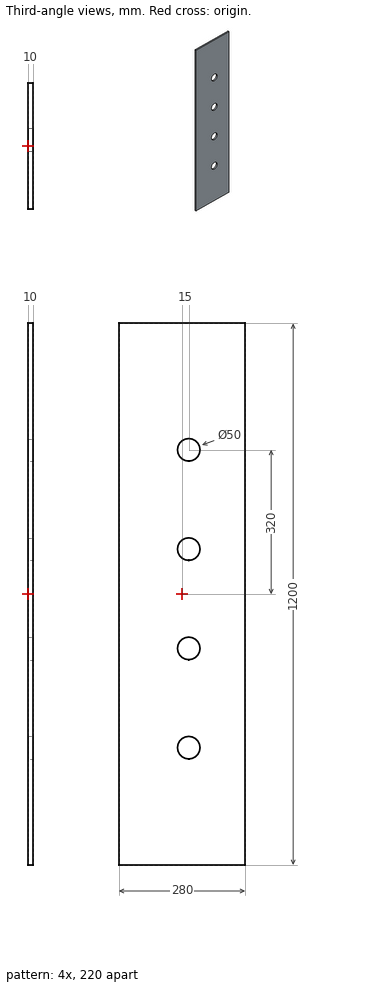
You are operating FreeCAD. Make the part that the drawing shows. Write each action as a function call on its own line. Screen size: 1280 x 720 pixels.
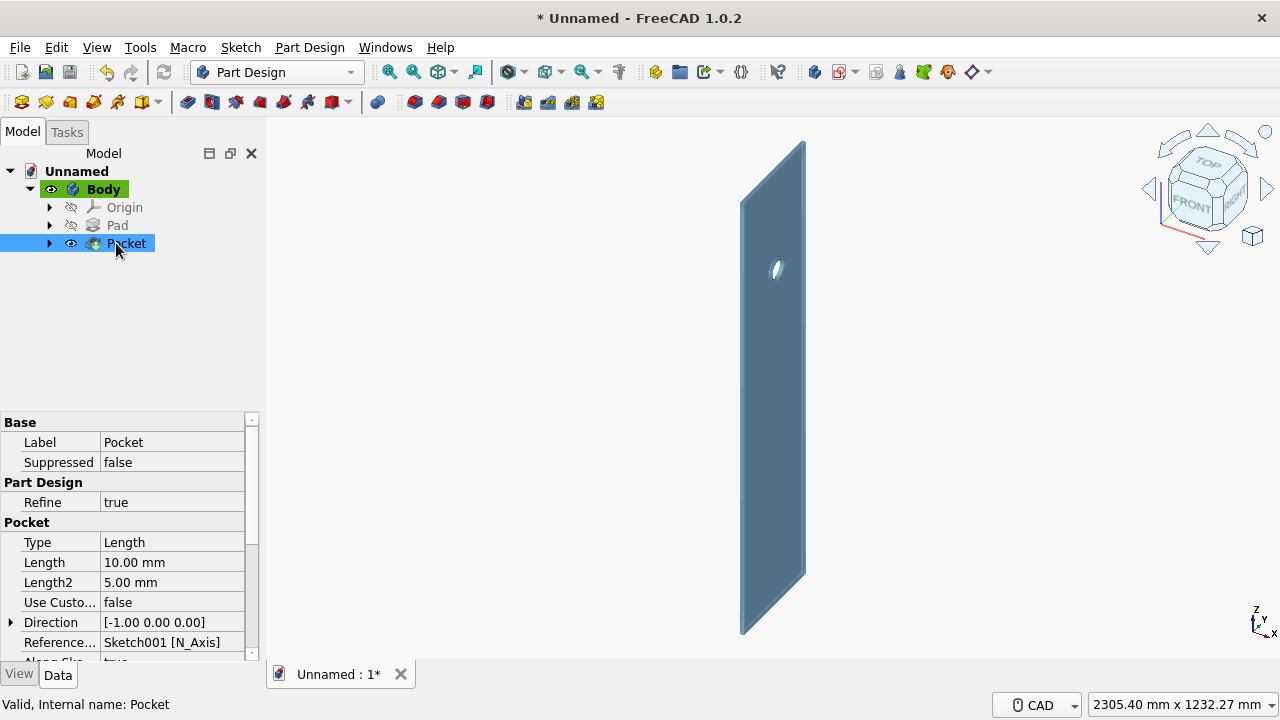
click(548, 102)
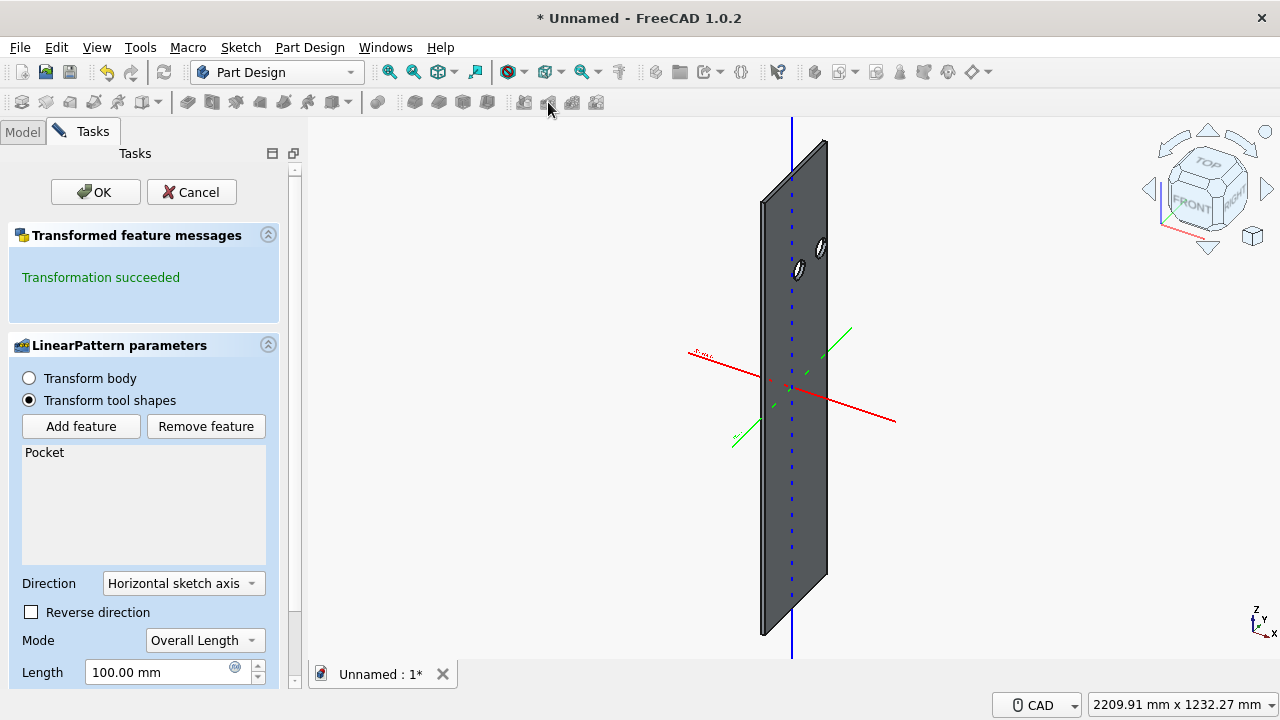
click(184, 584)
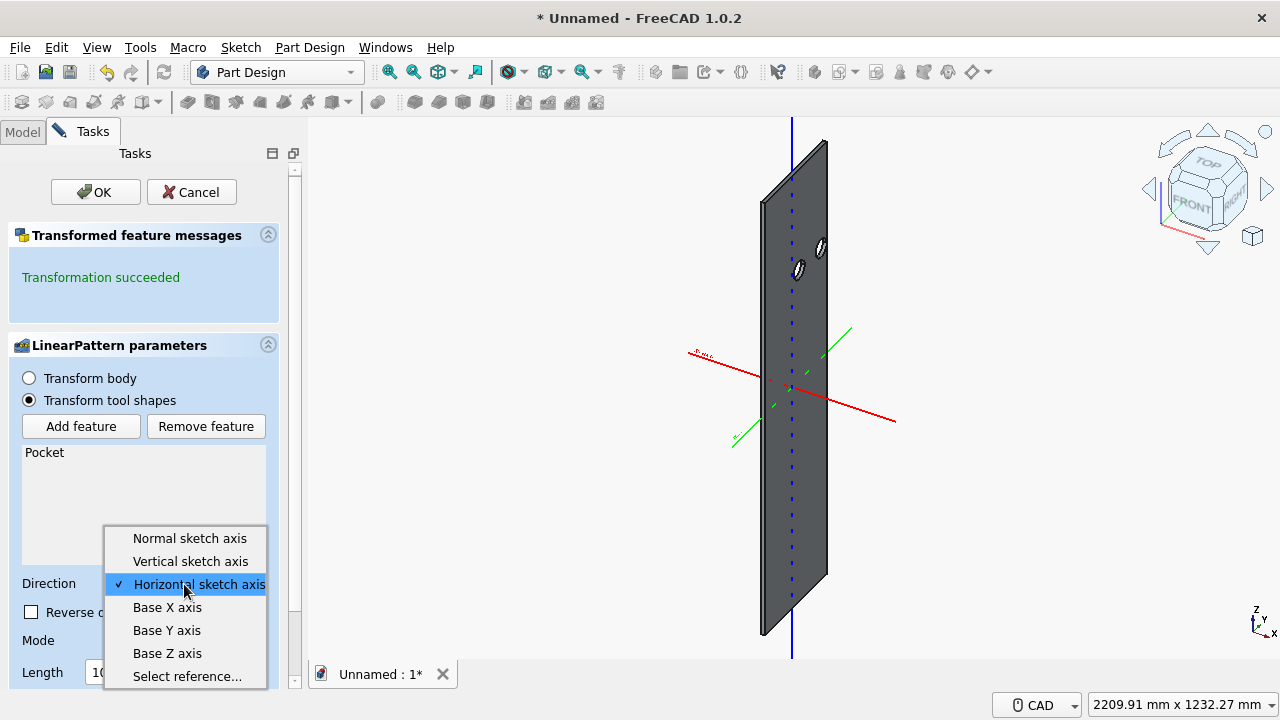
click(184, 654)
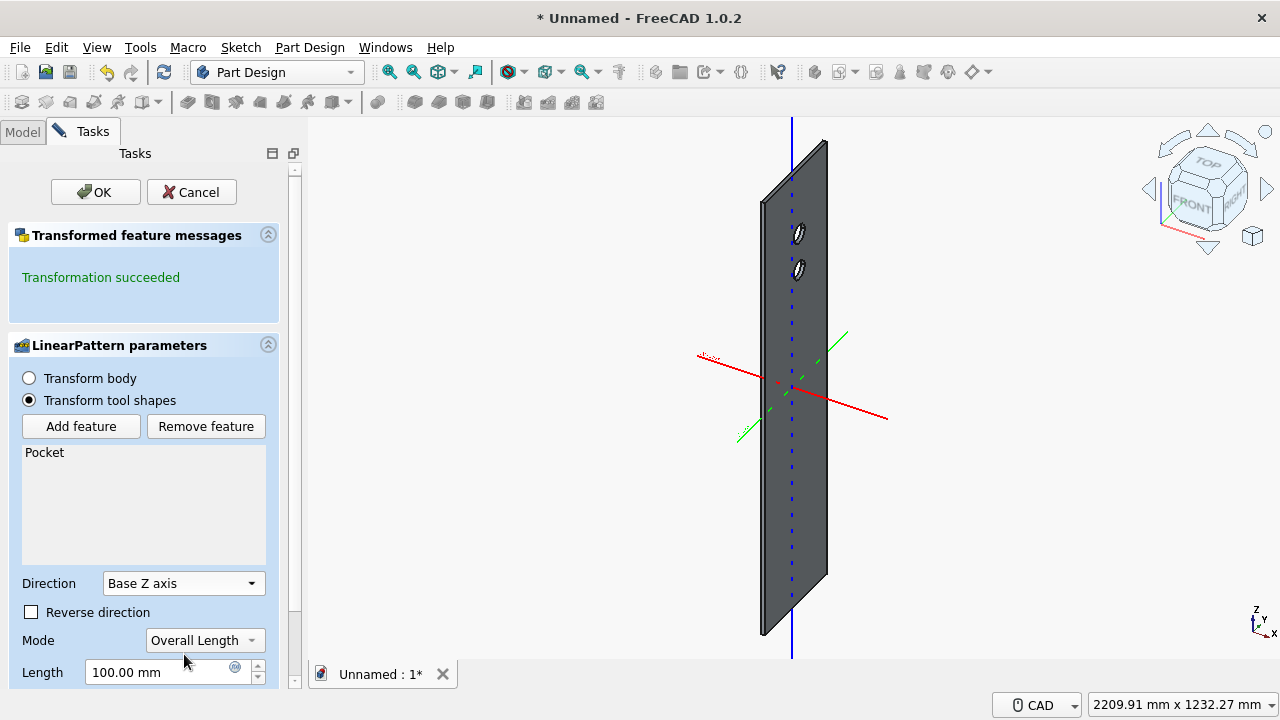
click(206, 640)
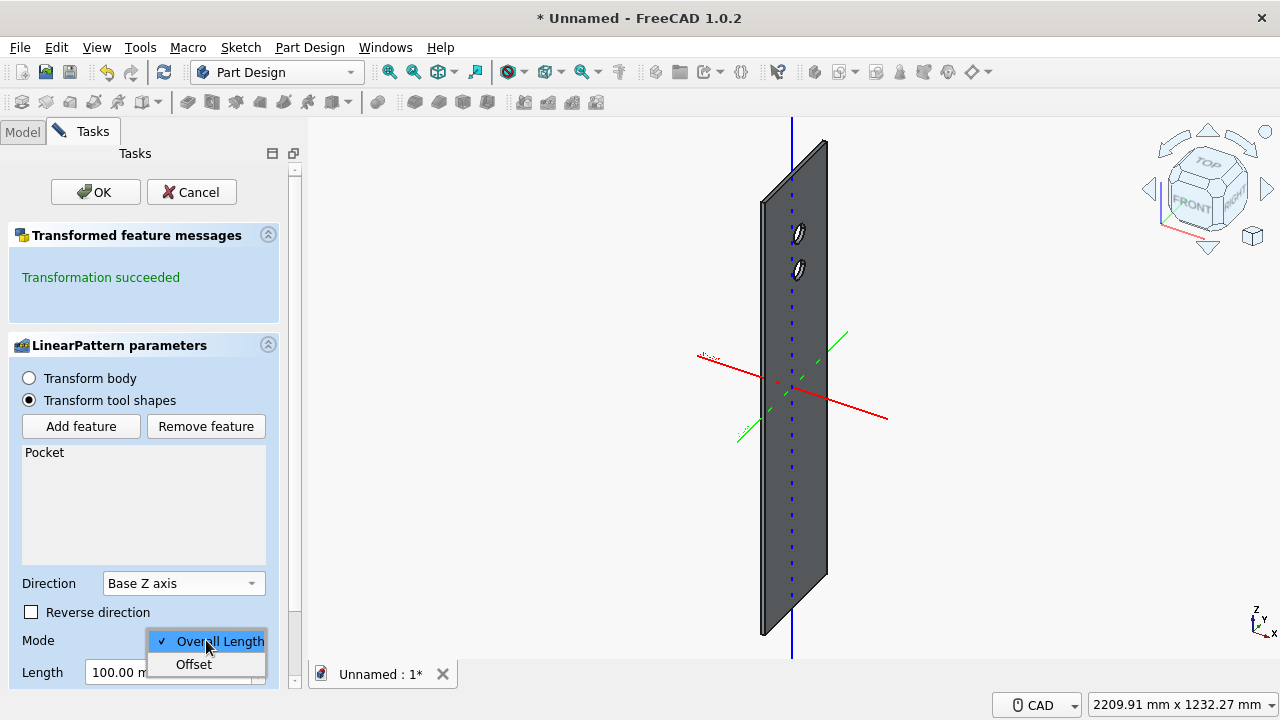
click(206, 664)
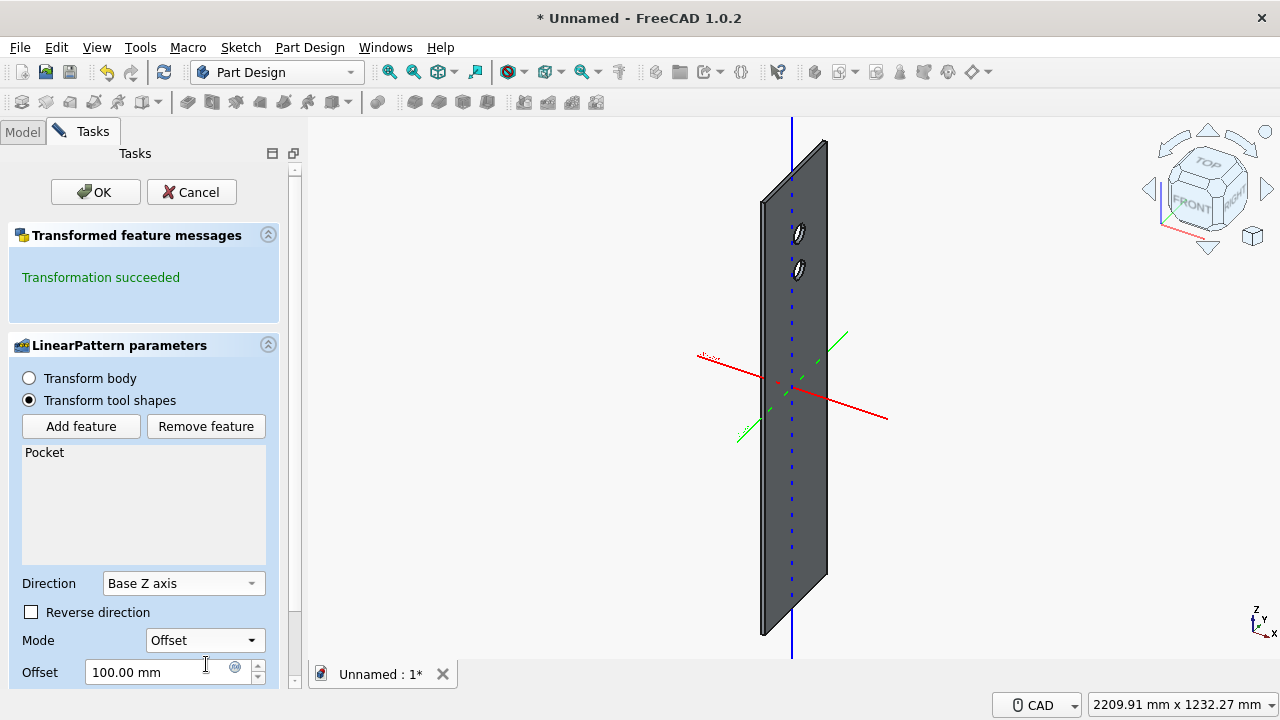
triple_click(168, 672)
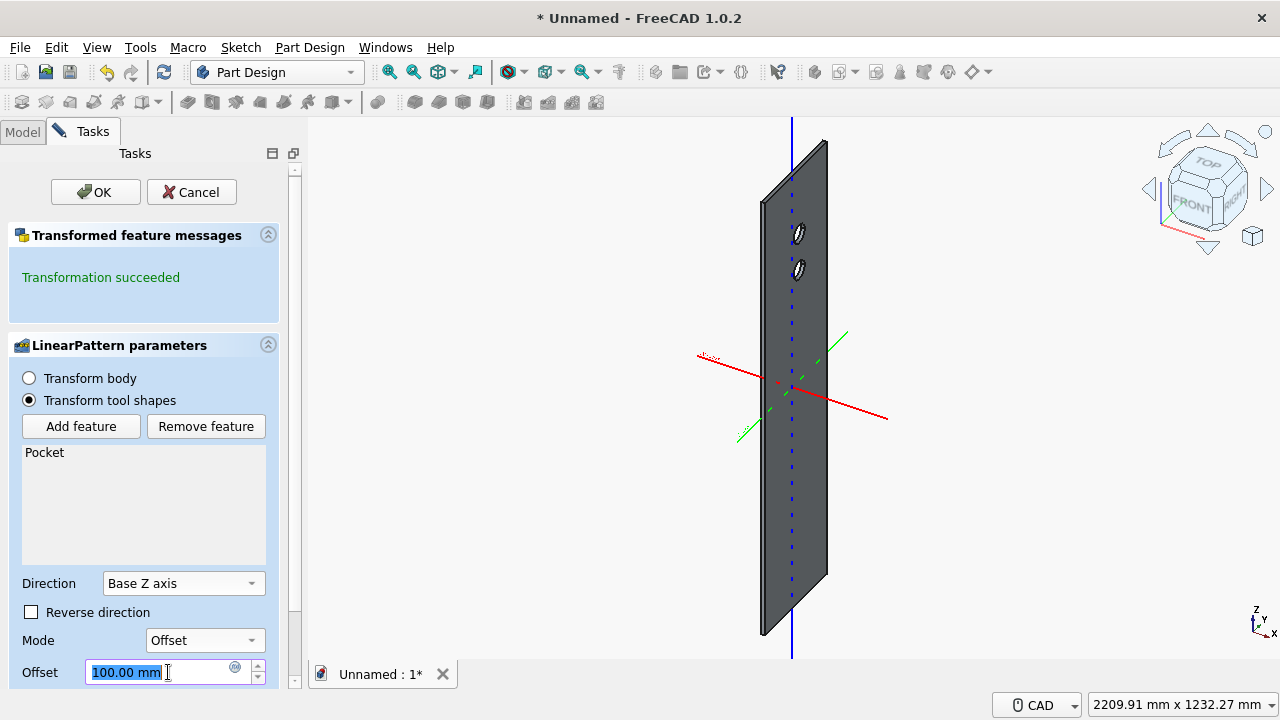
text(220)
key(Tab)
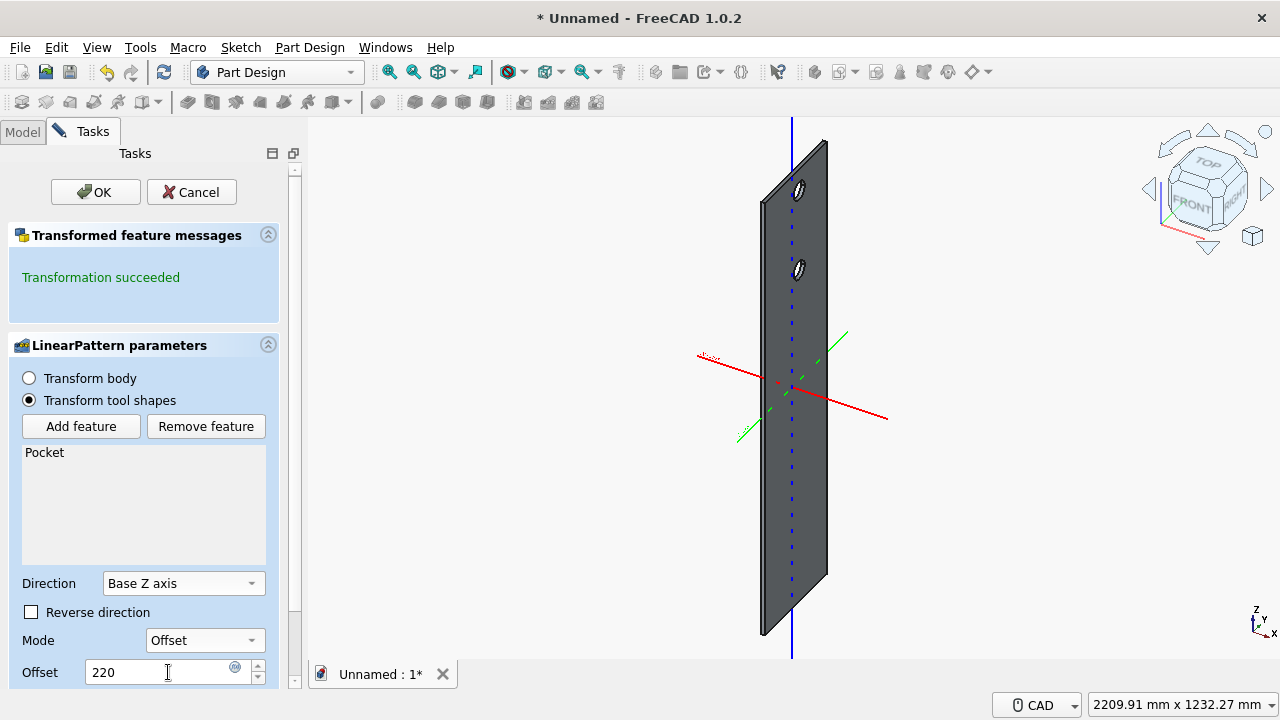
scroll(295, 426, down, 2)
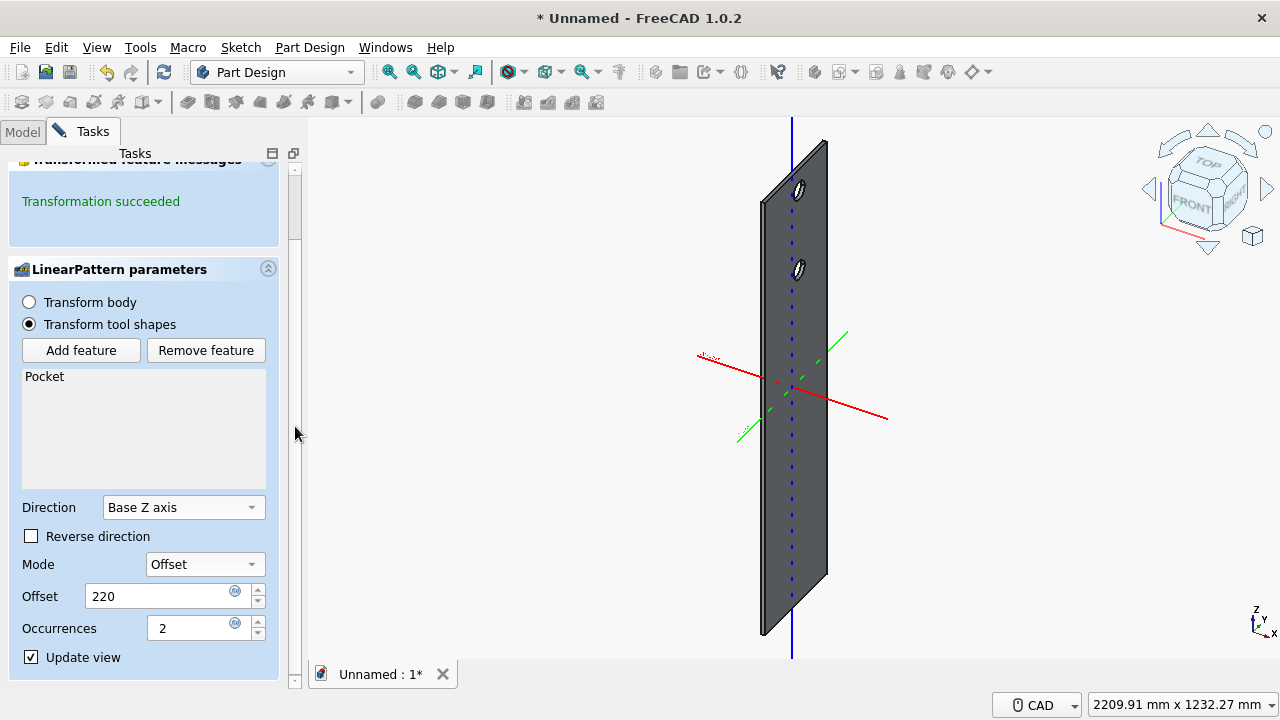
triple_click(198, 628)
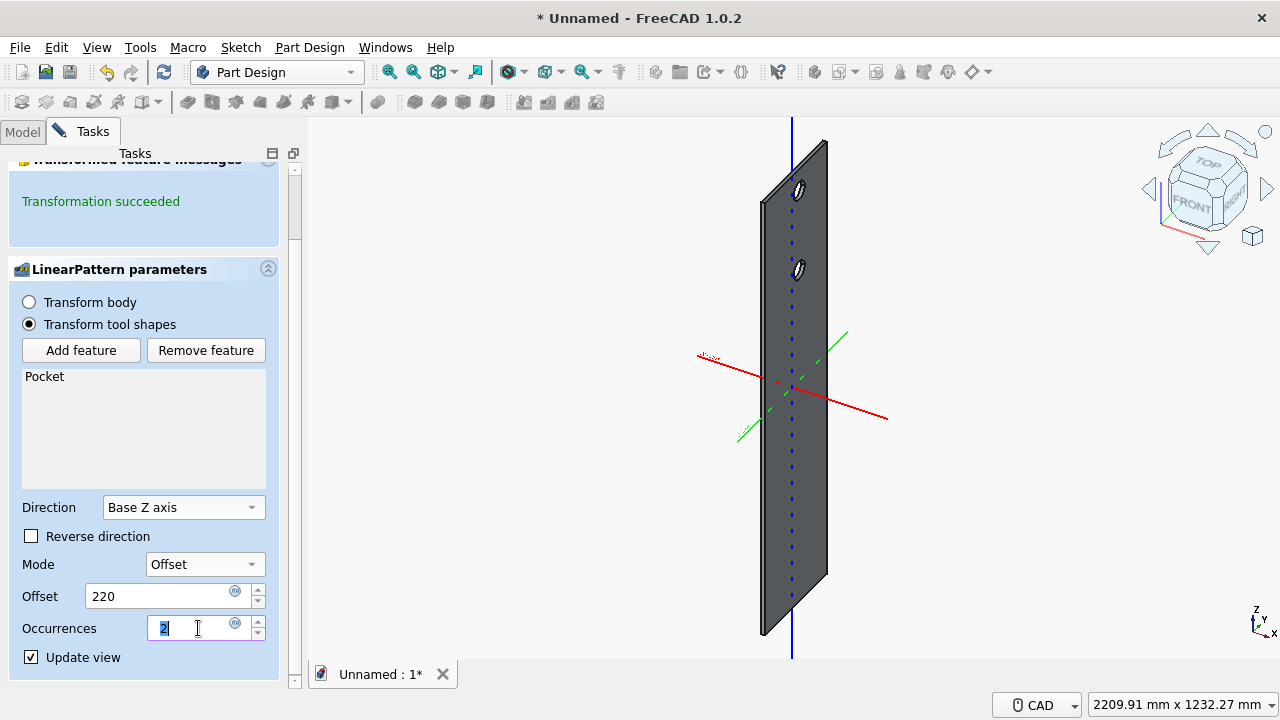
text(4)
key(Tab)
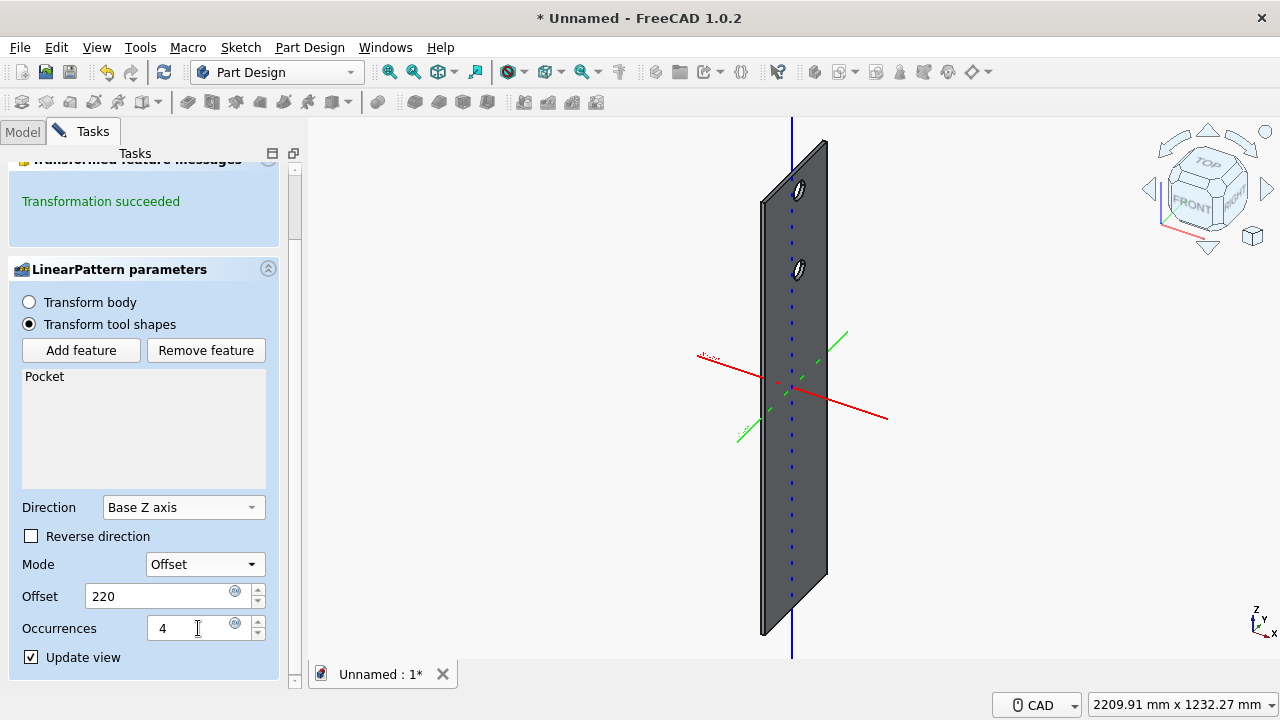
click(30, 536)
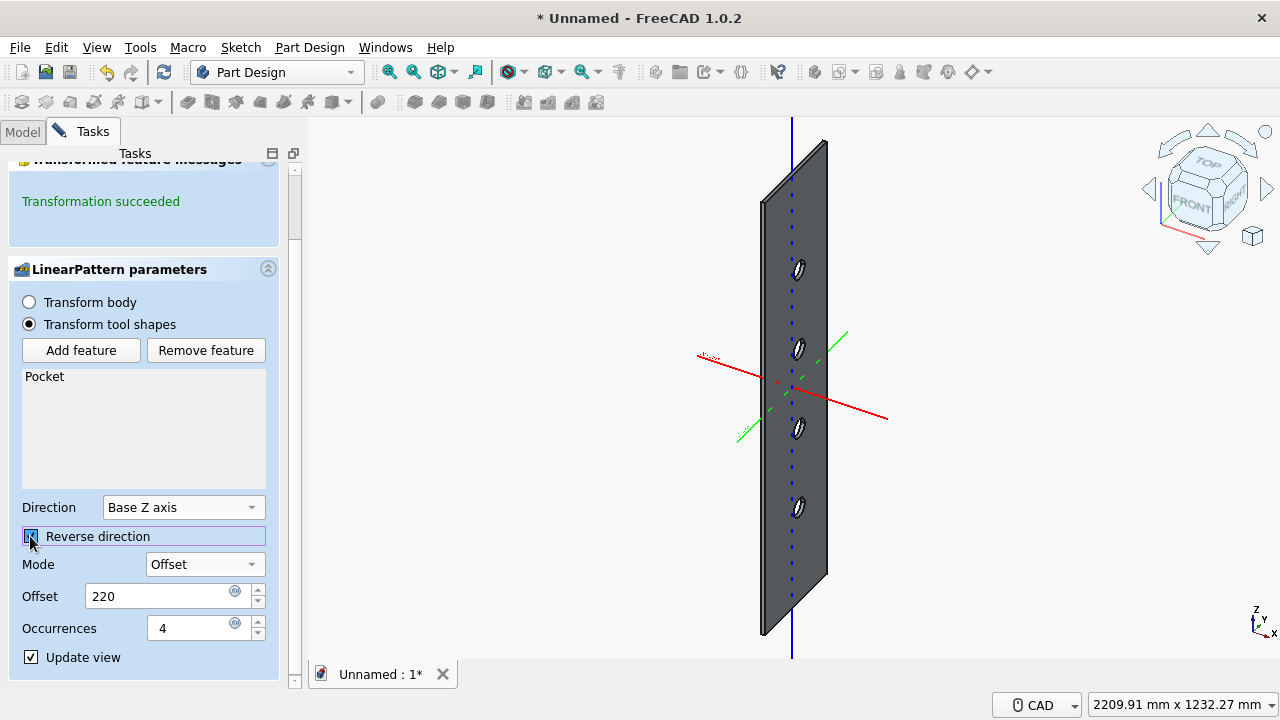
scroll(295, 426, up, 3)